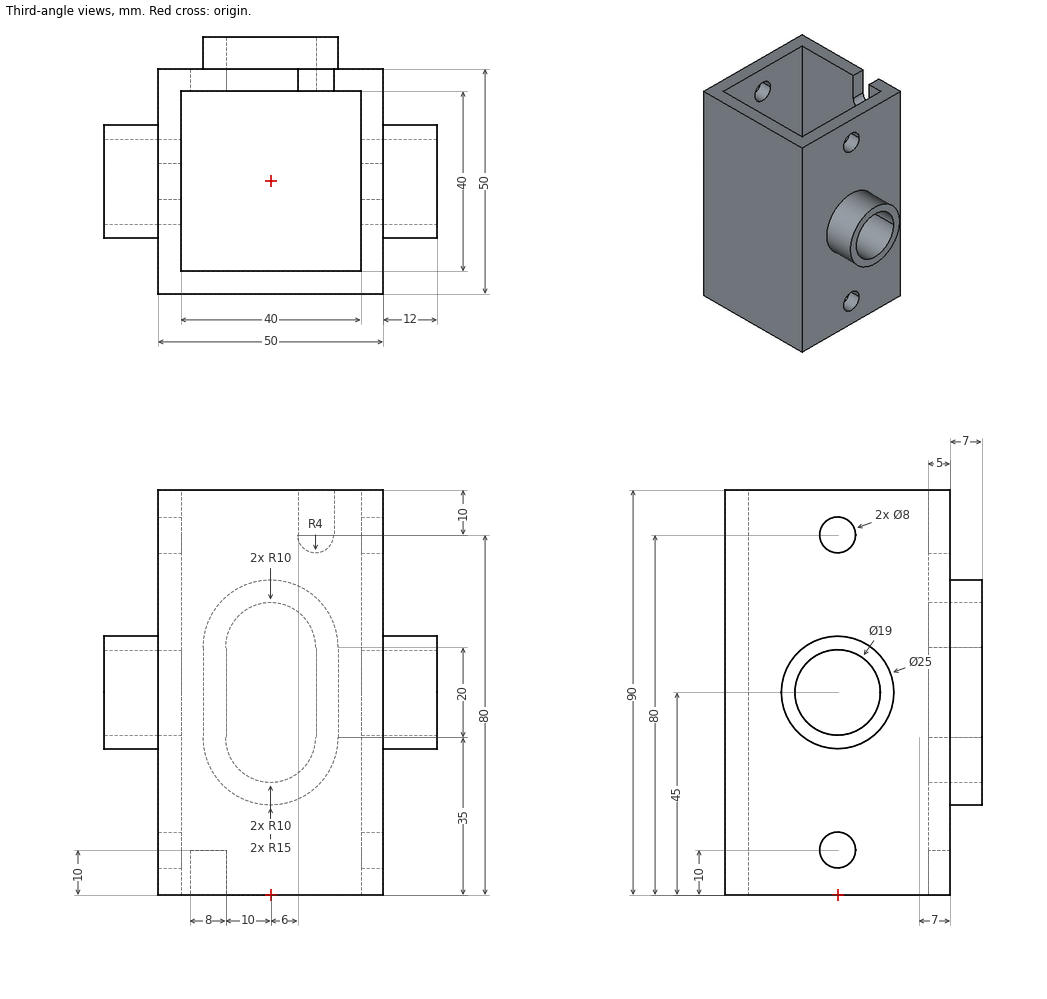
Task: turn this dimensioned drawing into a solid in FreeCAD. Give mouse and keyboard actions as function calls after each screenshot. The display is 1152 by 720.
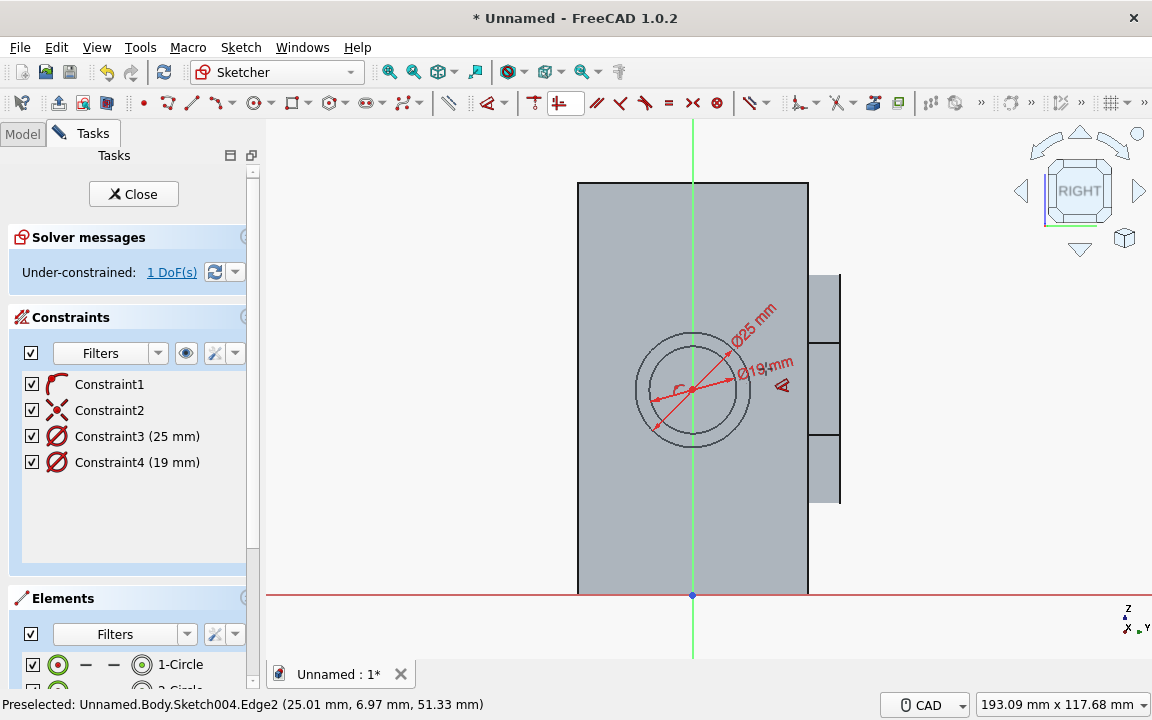
click(693, 390)
click(727, 493)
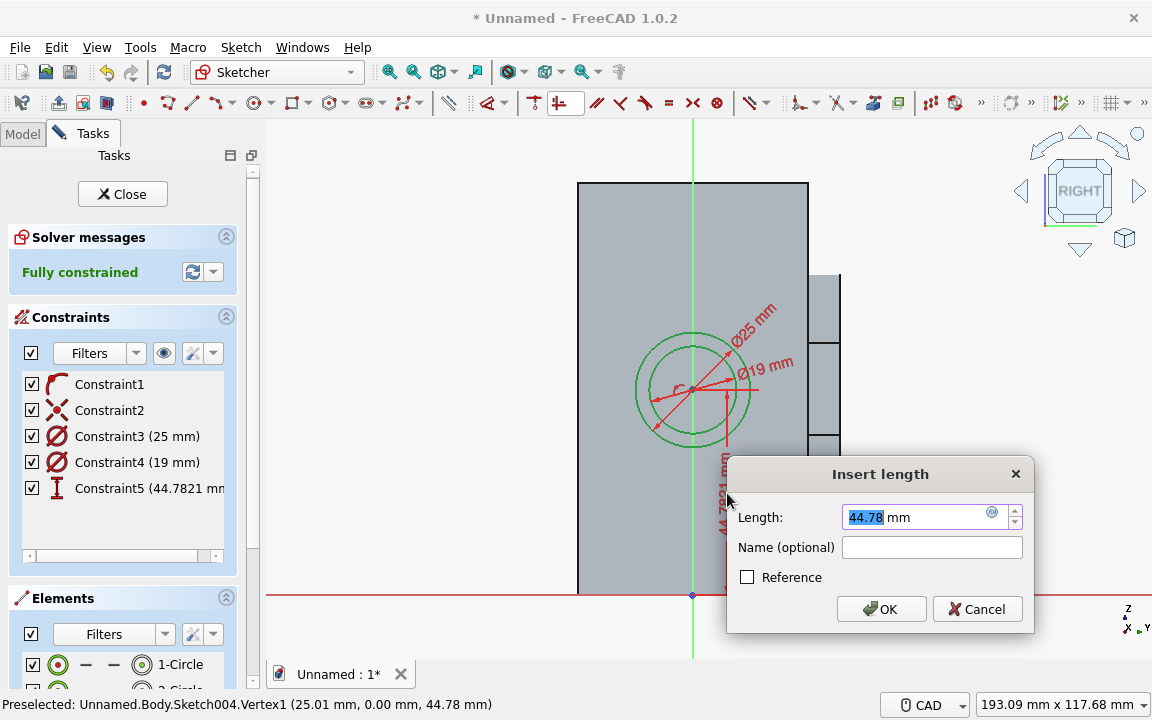
text(45)
key(Return)
key(Escape)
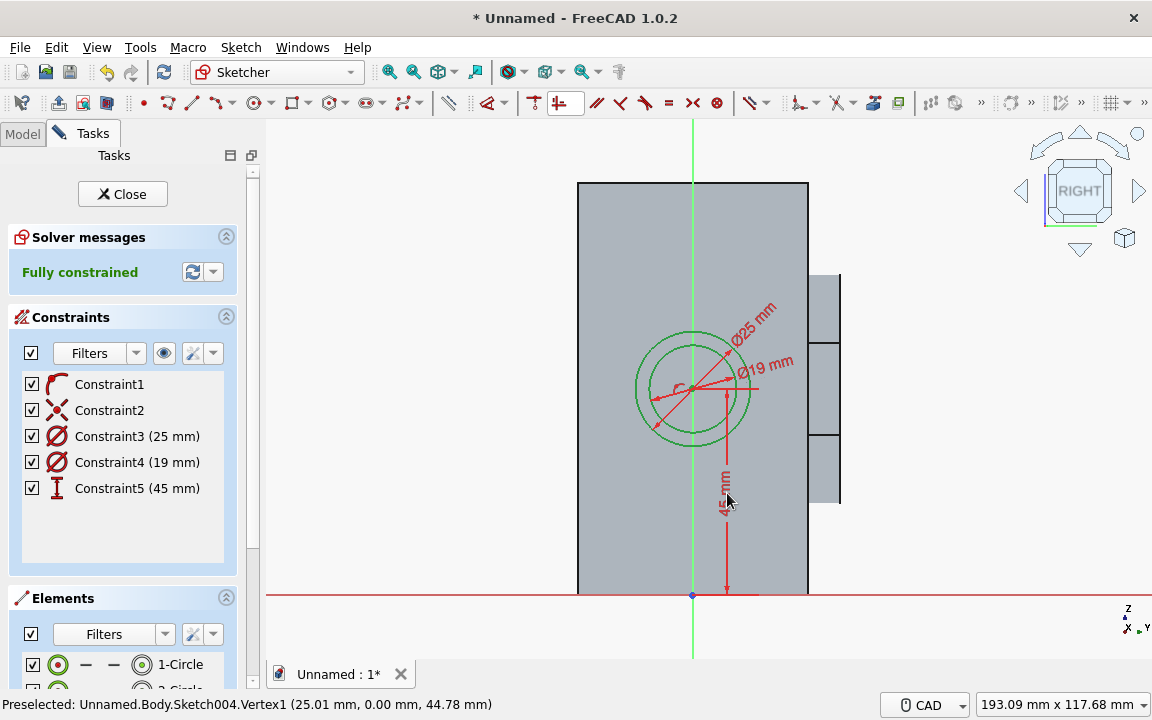
click(123, 194)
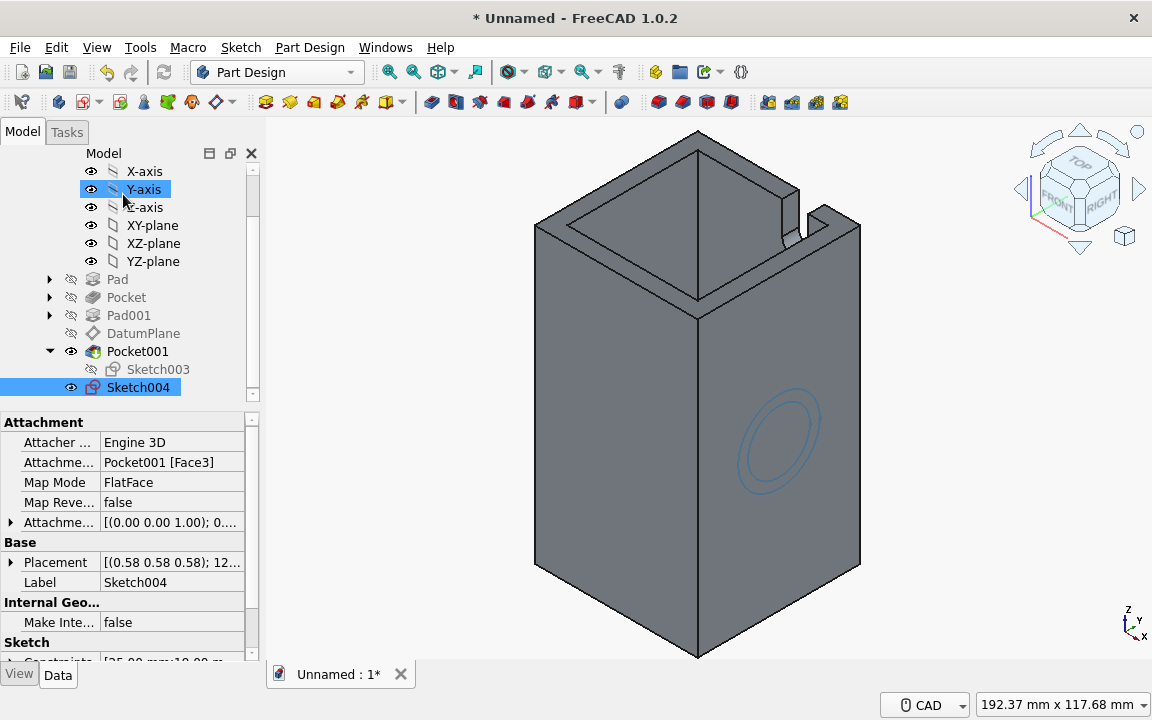
click(266, 102)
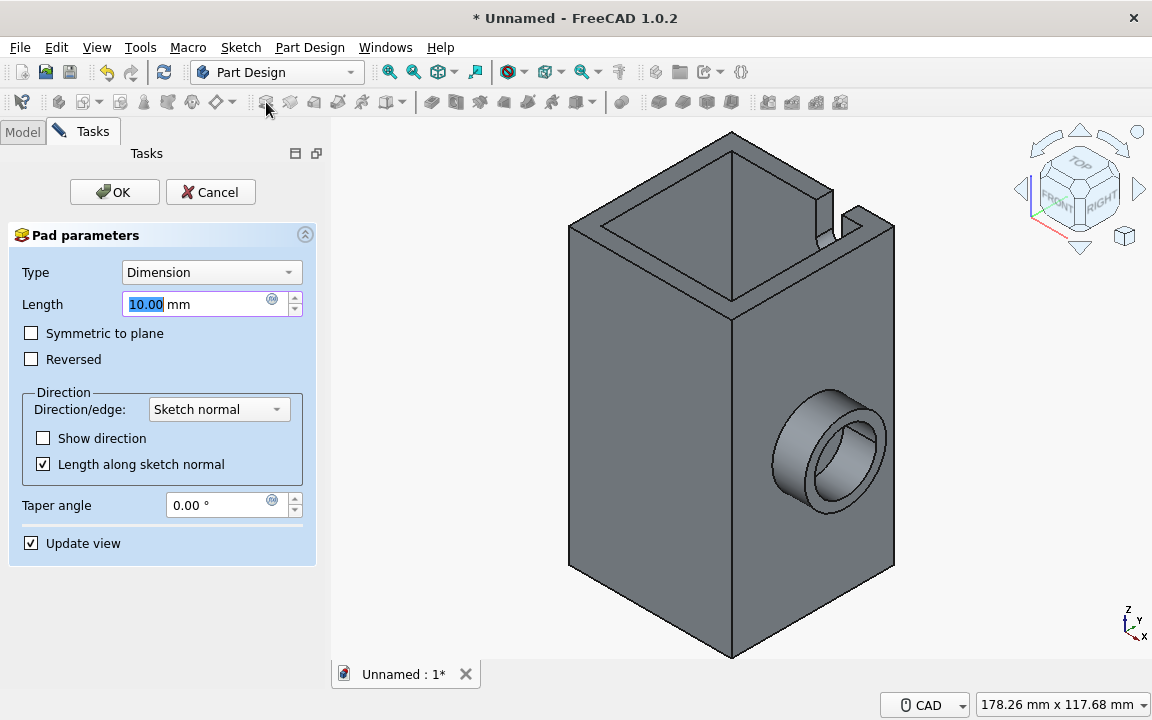
text(12)
key(Tab)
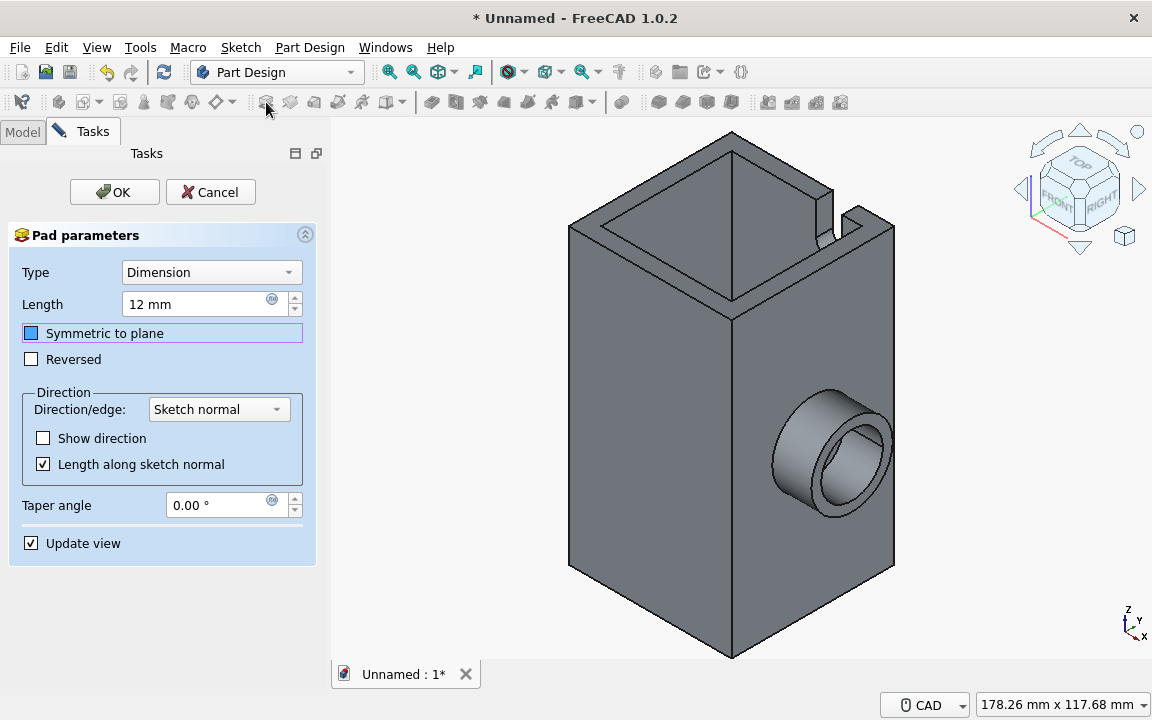
click(115, 192)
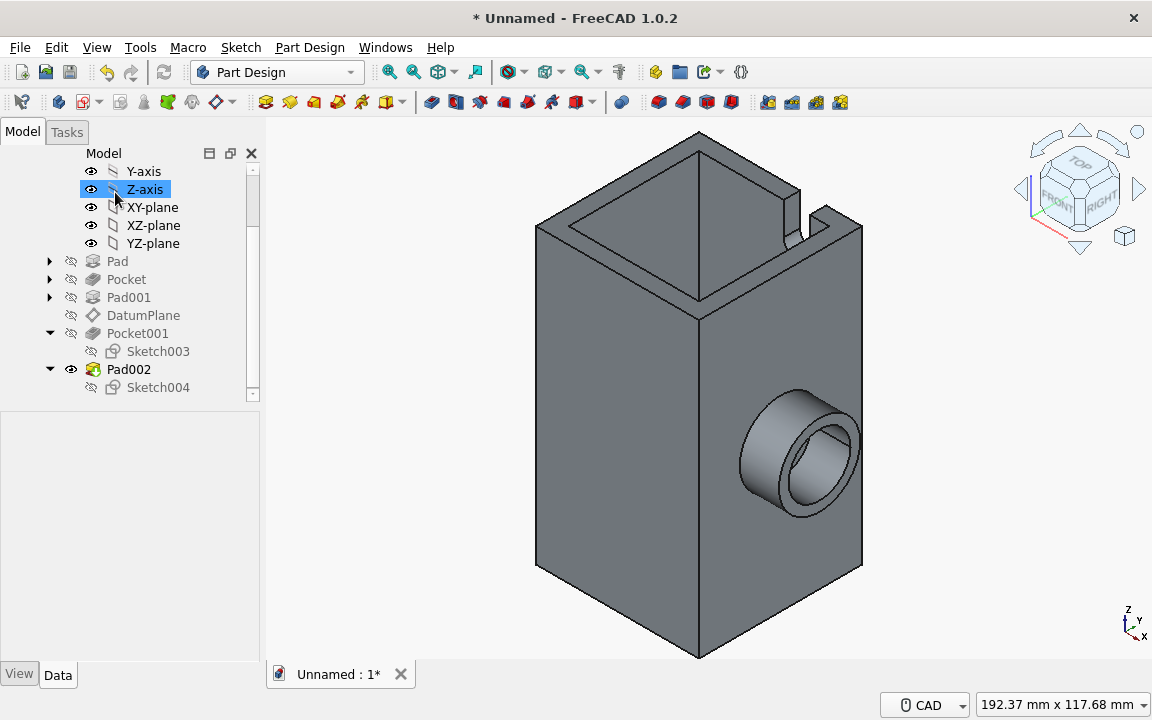
click(390, 72)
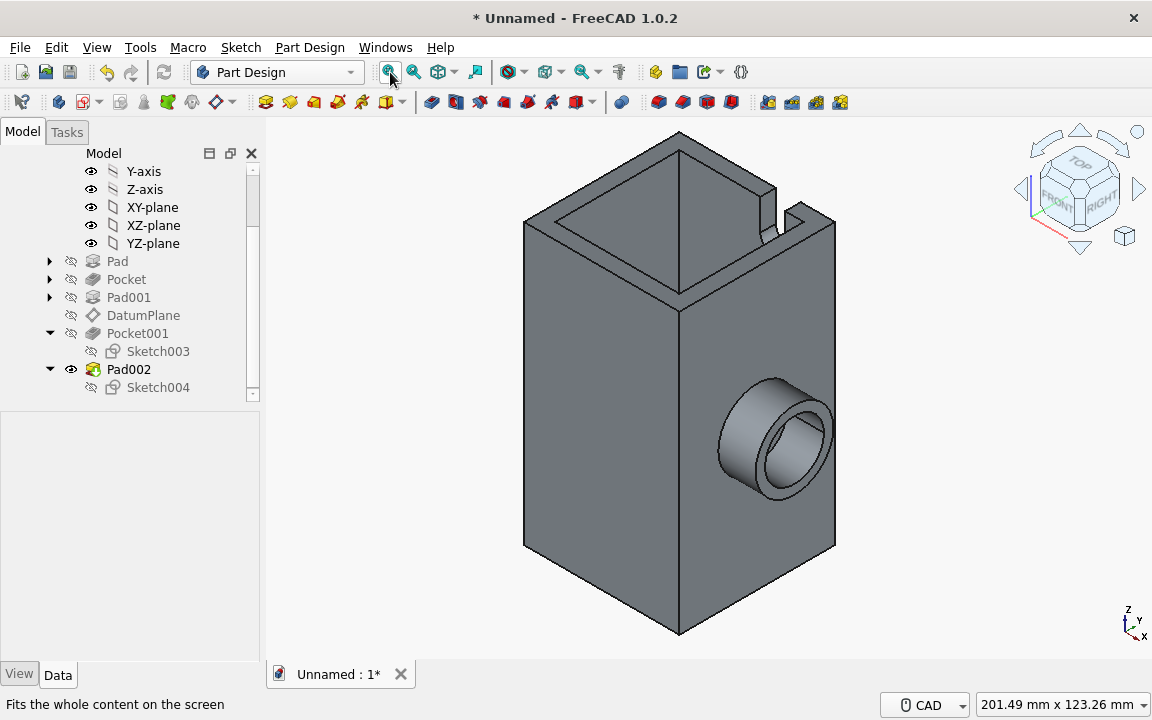
click(779, 322)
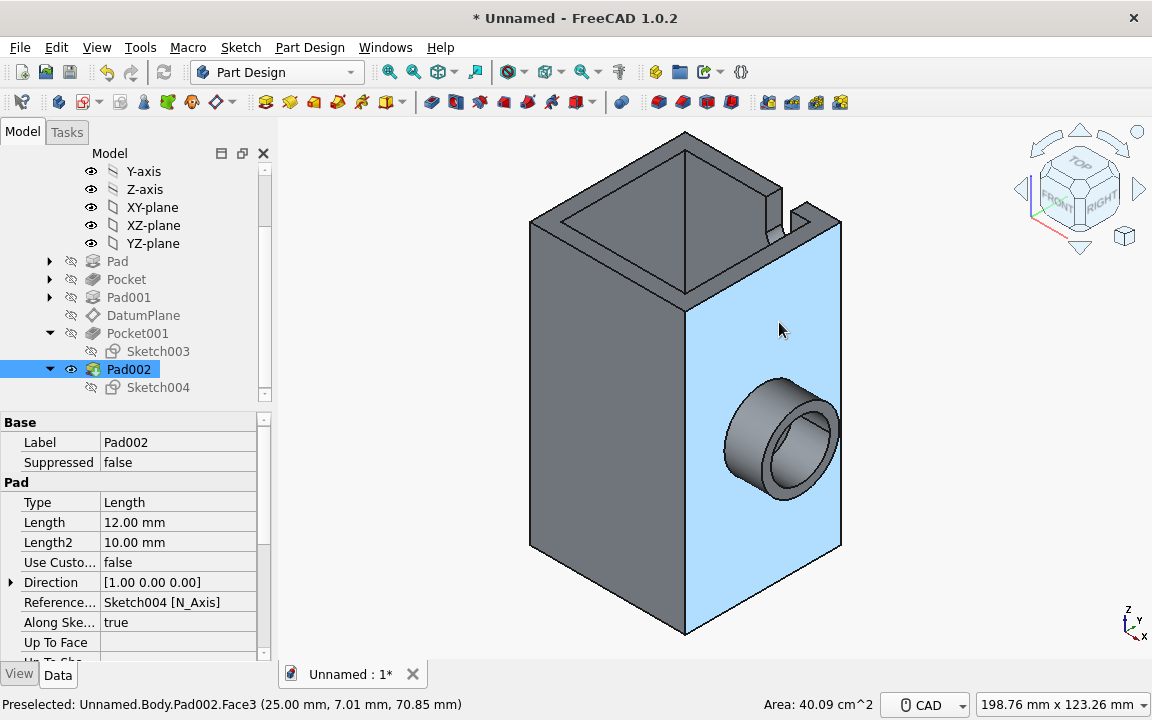
click(84, 102)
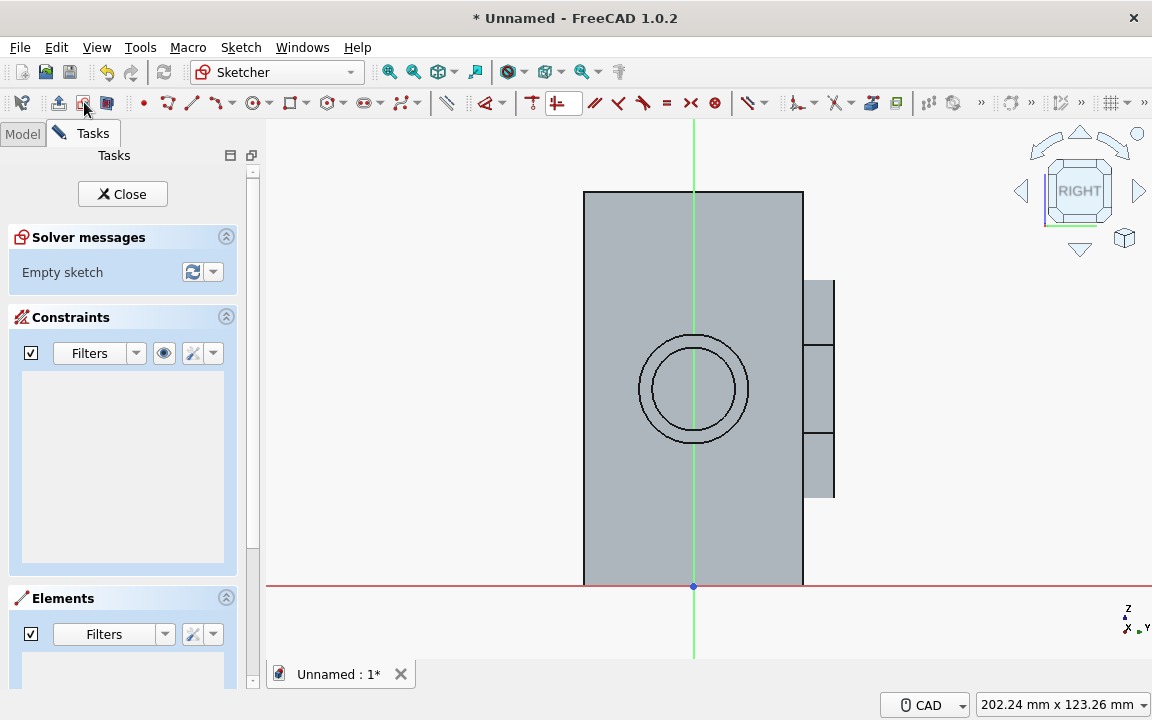
click(254, 104)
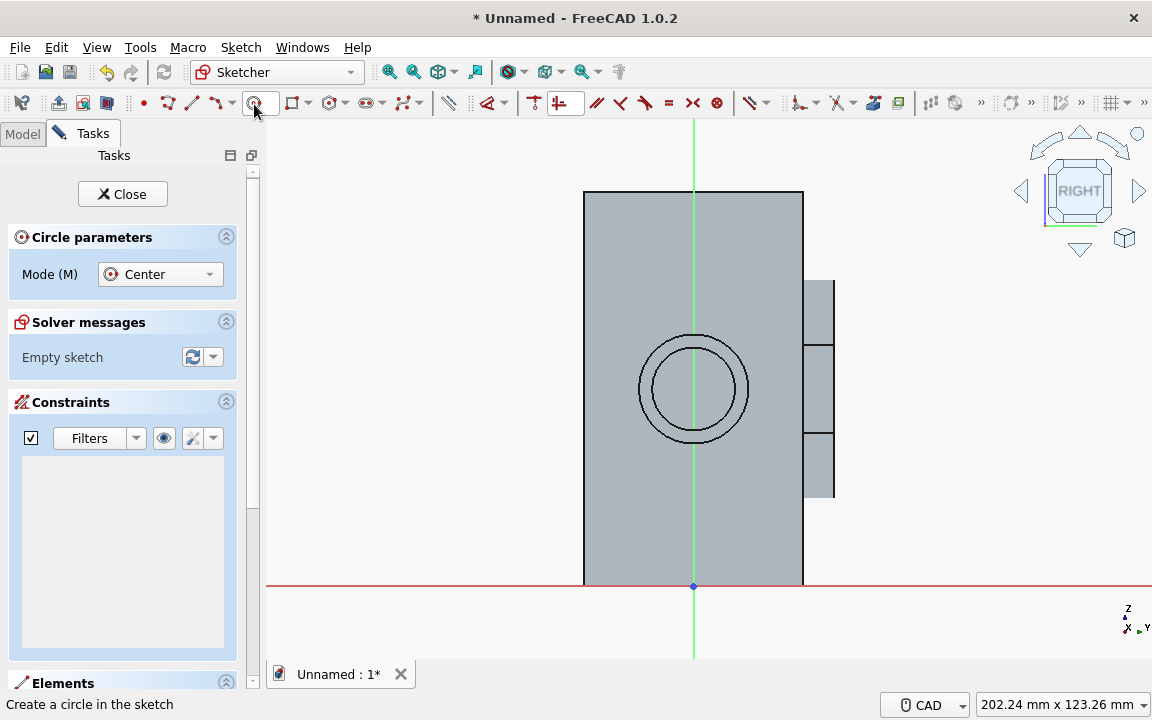
scroll(694, 236, up, 2)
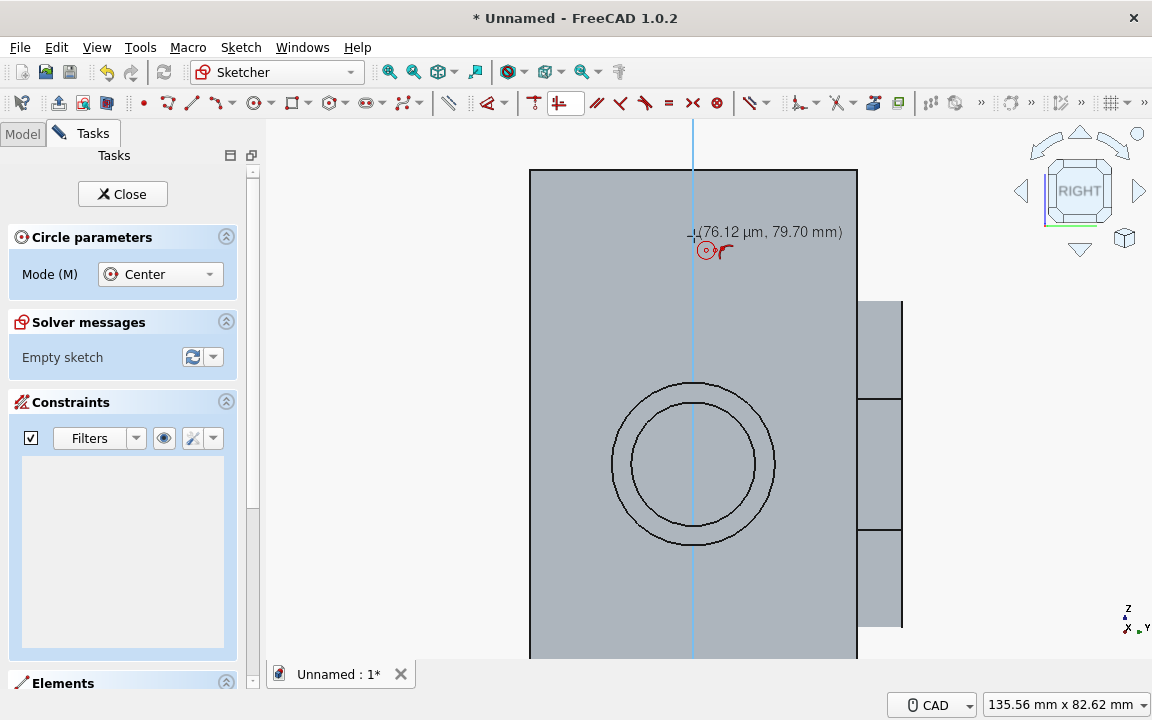
click(693, 235)
click(712, 217)